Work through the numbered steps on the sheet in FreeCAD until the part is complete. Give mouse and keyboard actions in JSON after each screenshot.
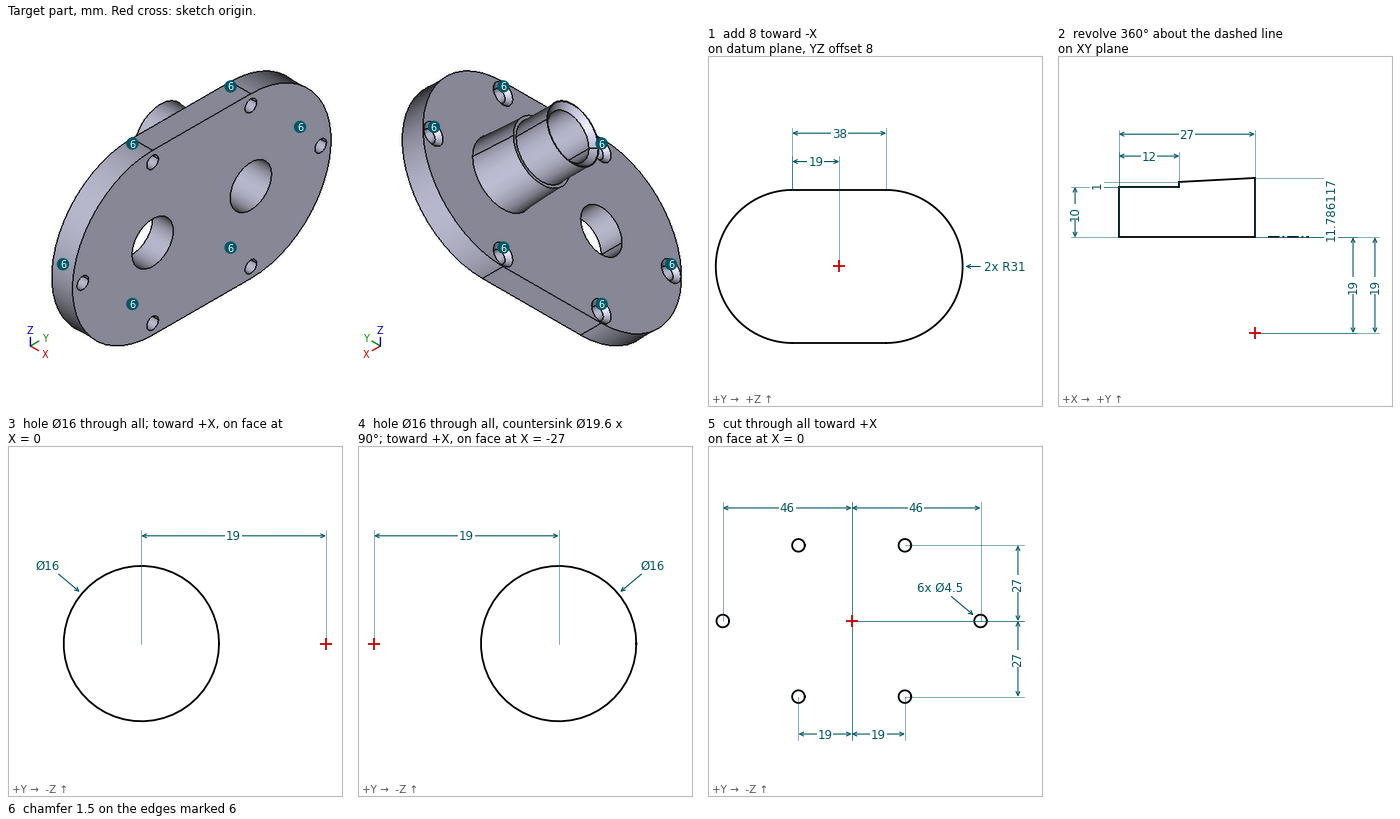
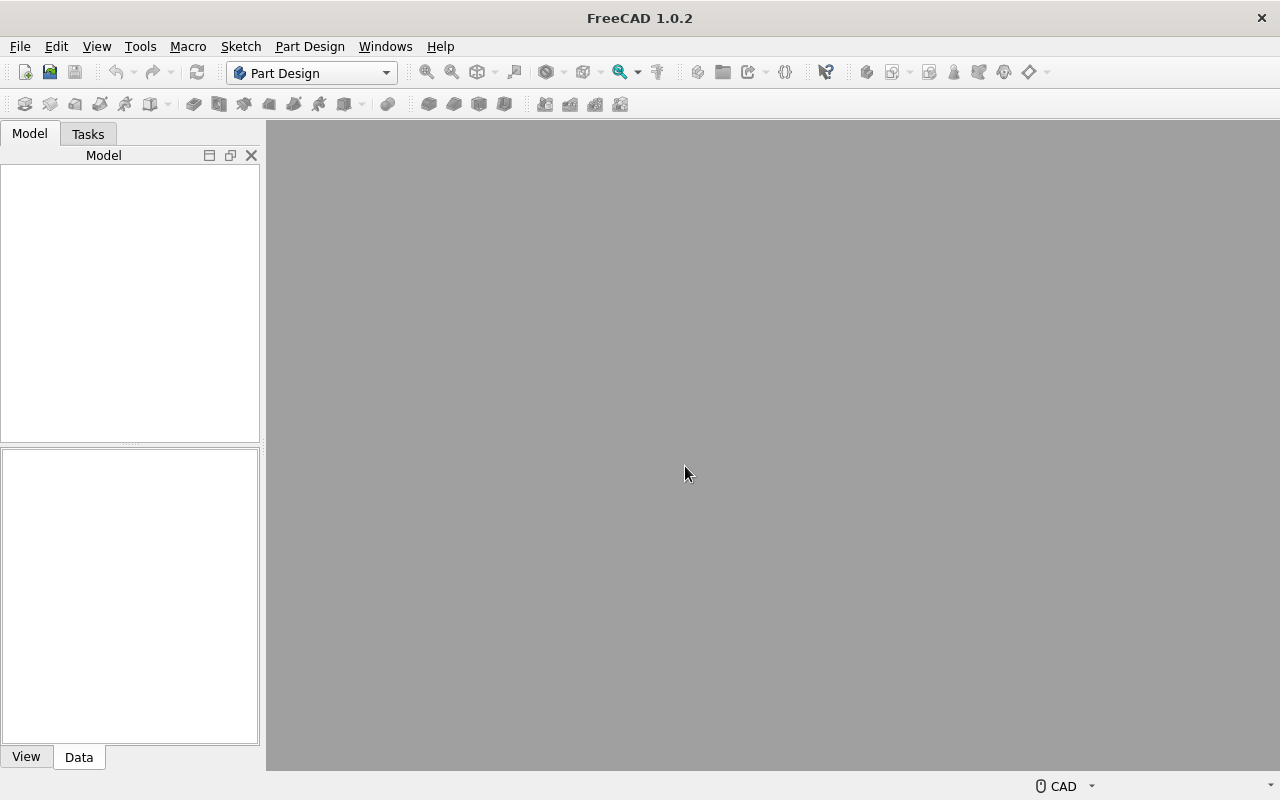
{"action": "key", "text": "ctrl+n"}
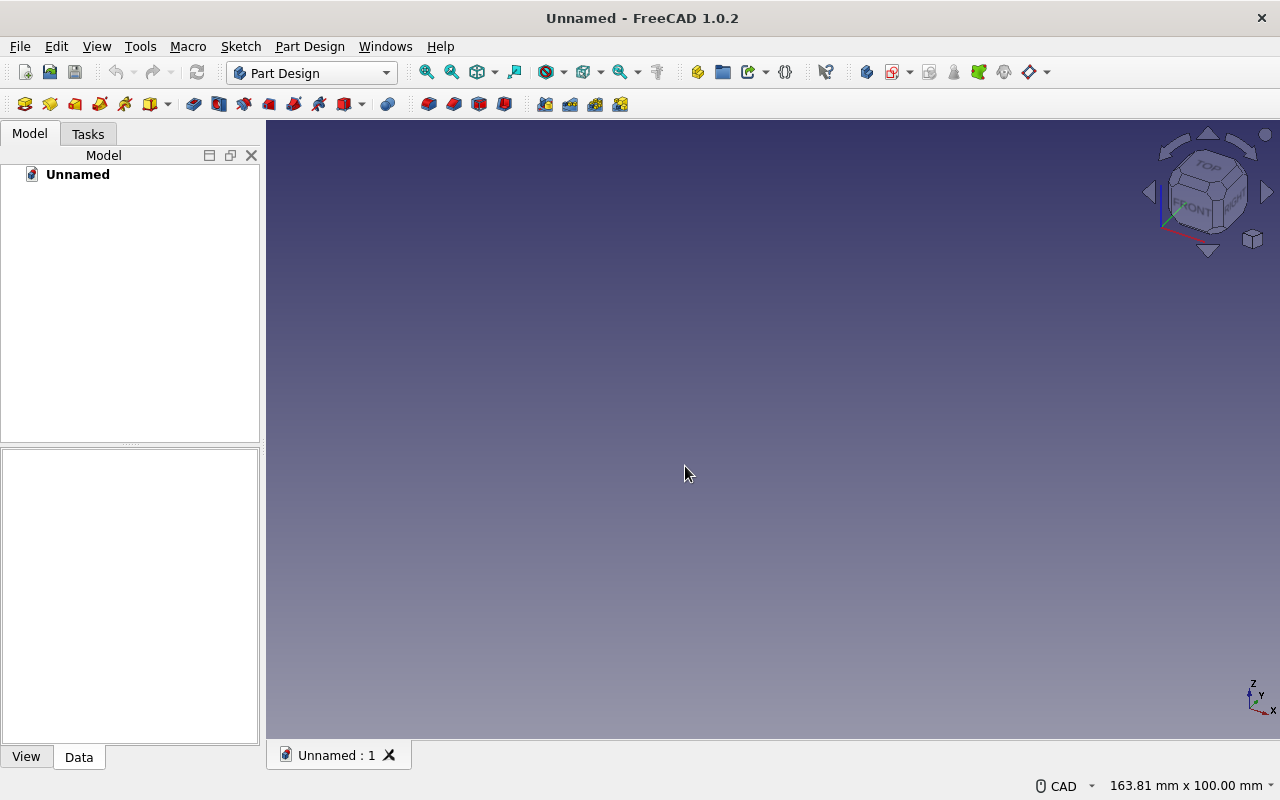
{"action": "left_click", "coordinate": [867, 72]}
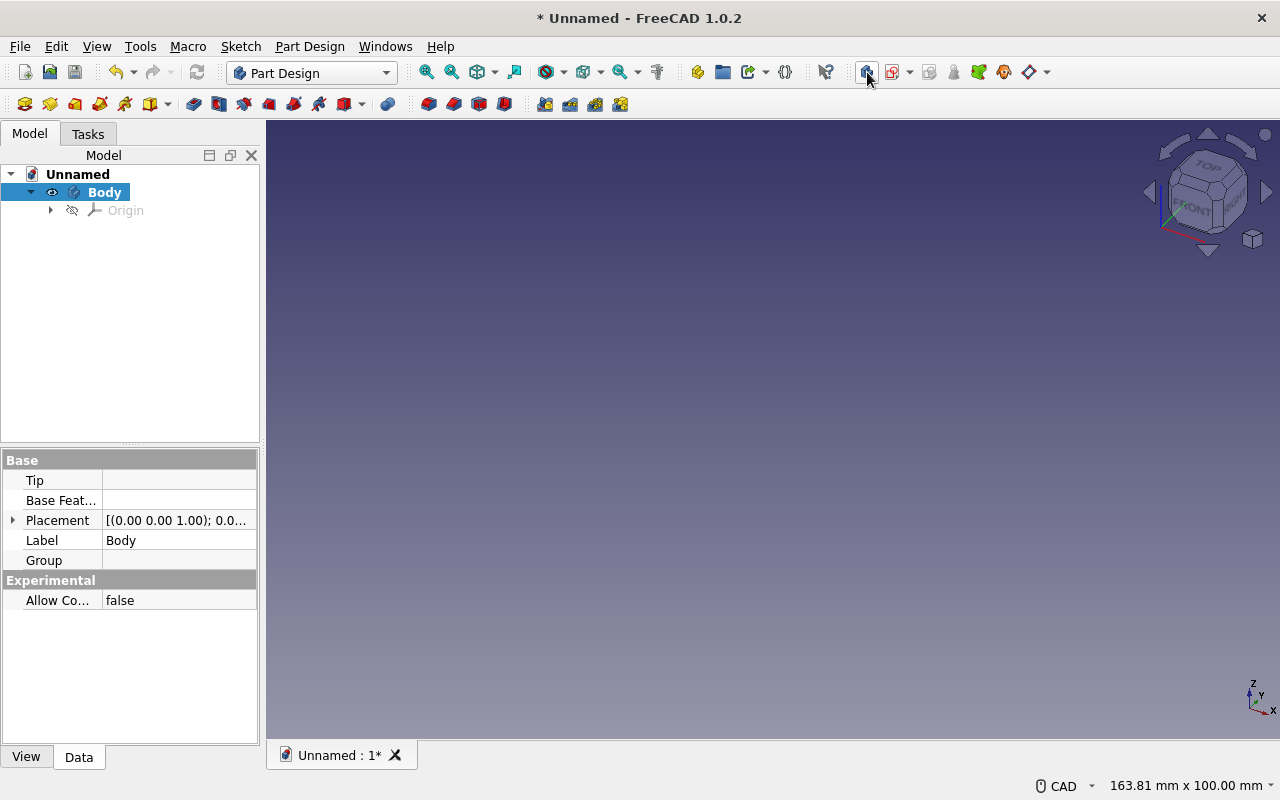
{"action": "left_click", "coordinate": [51, 210]}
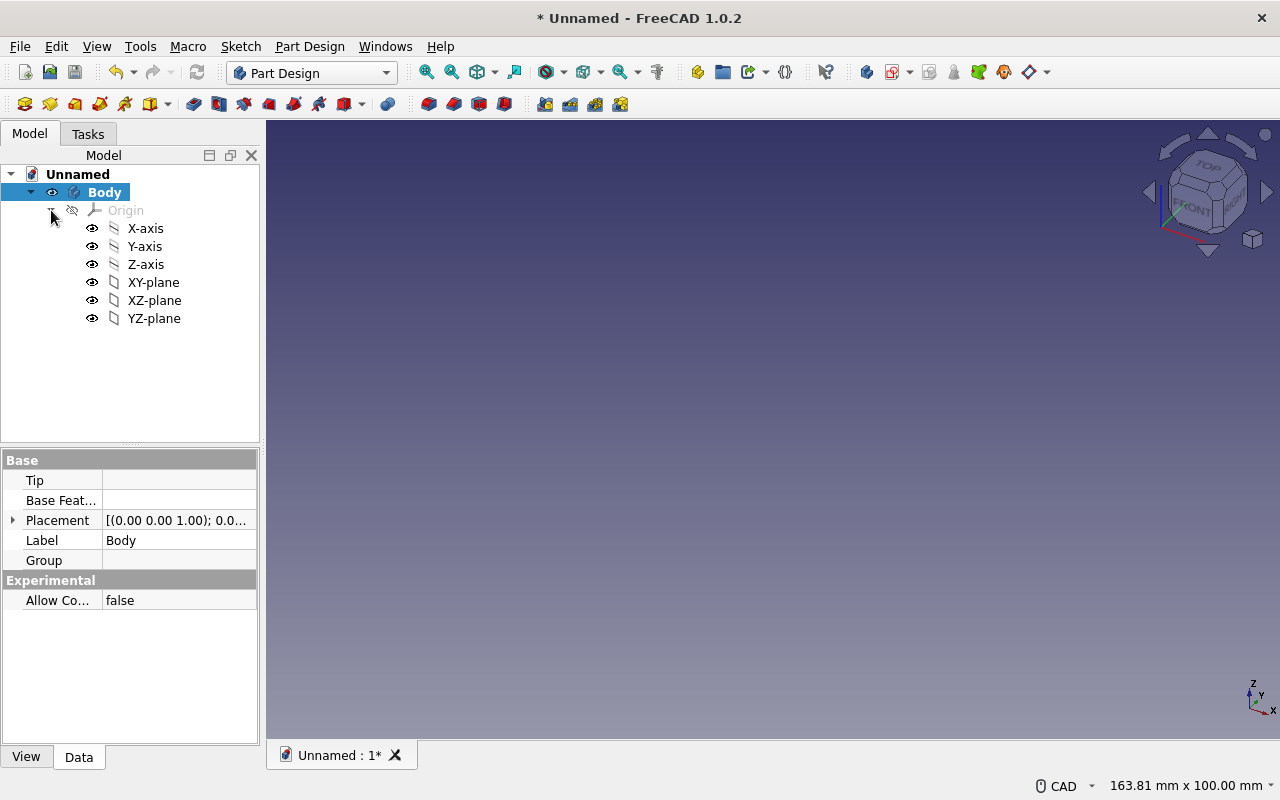
{"action": "left_click", "coordinate": [137, 318]}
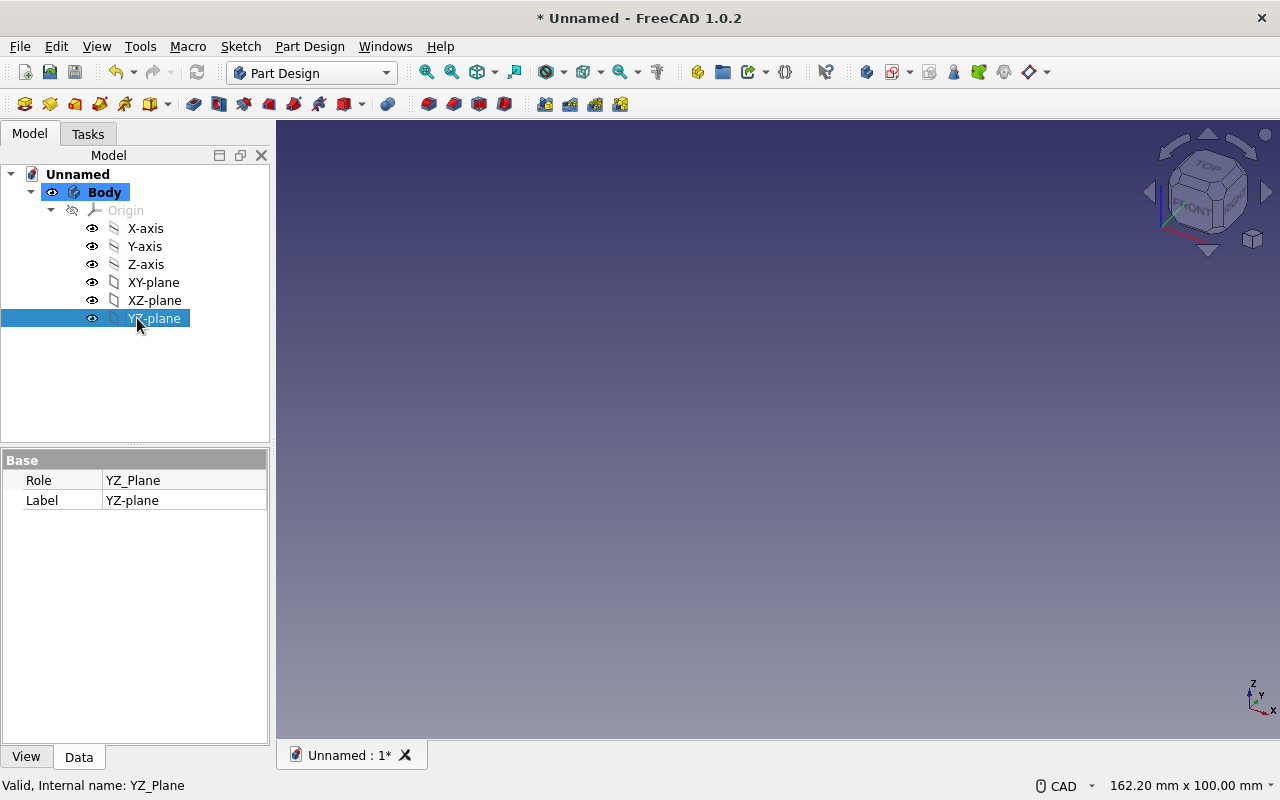
{"action": "left_click", "coordinate": [1028, 72]}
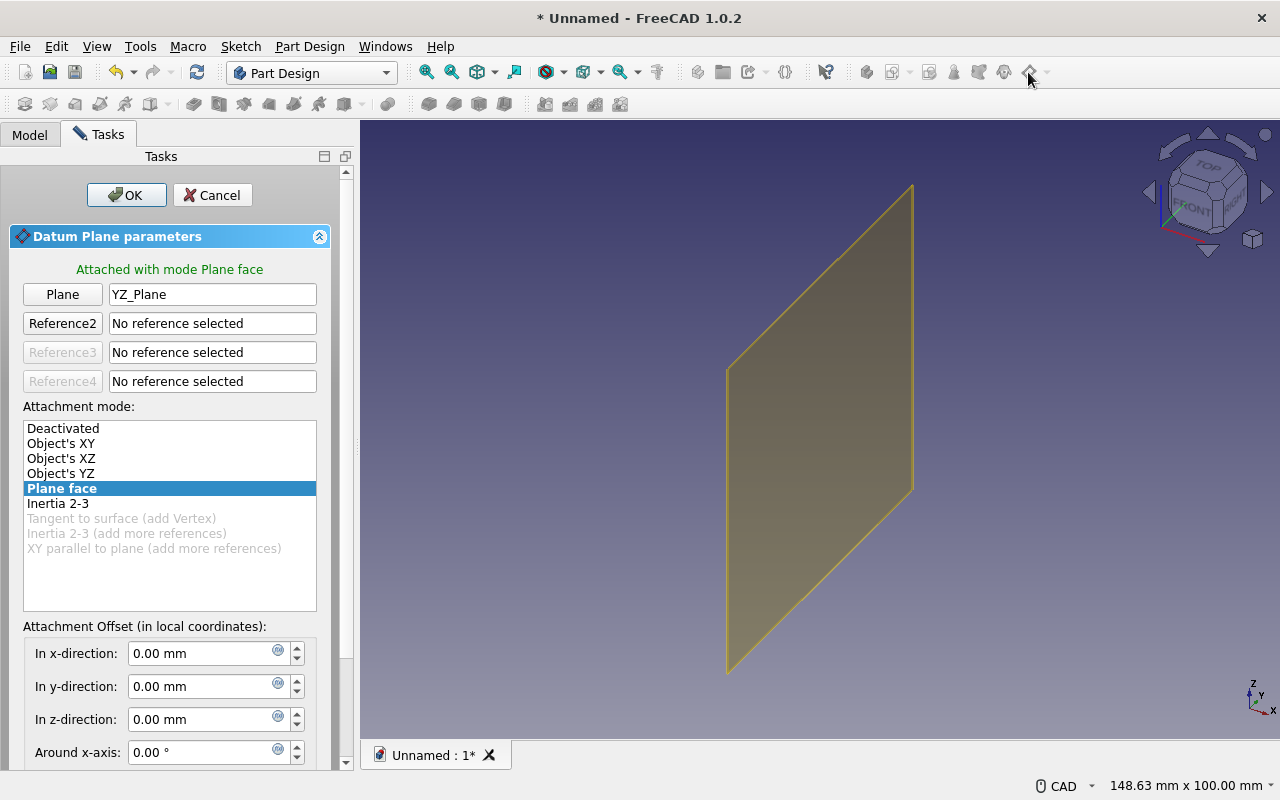
{"action": "triple_click", "coordinate": [210, 720]}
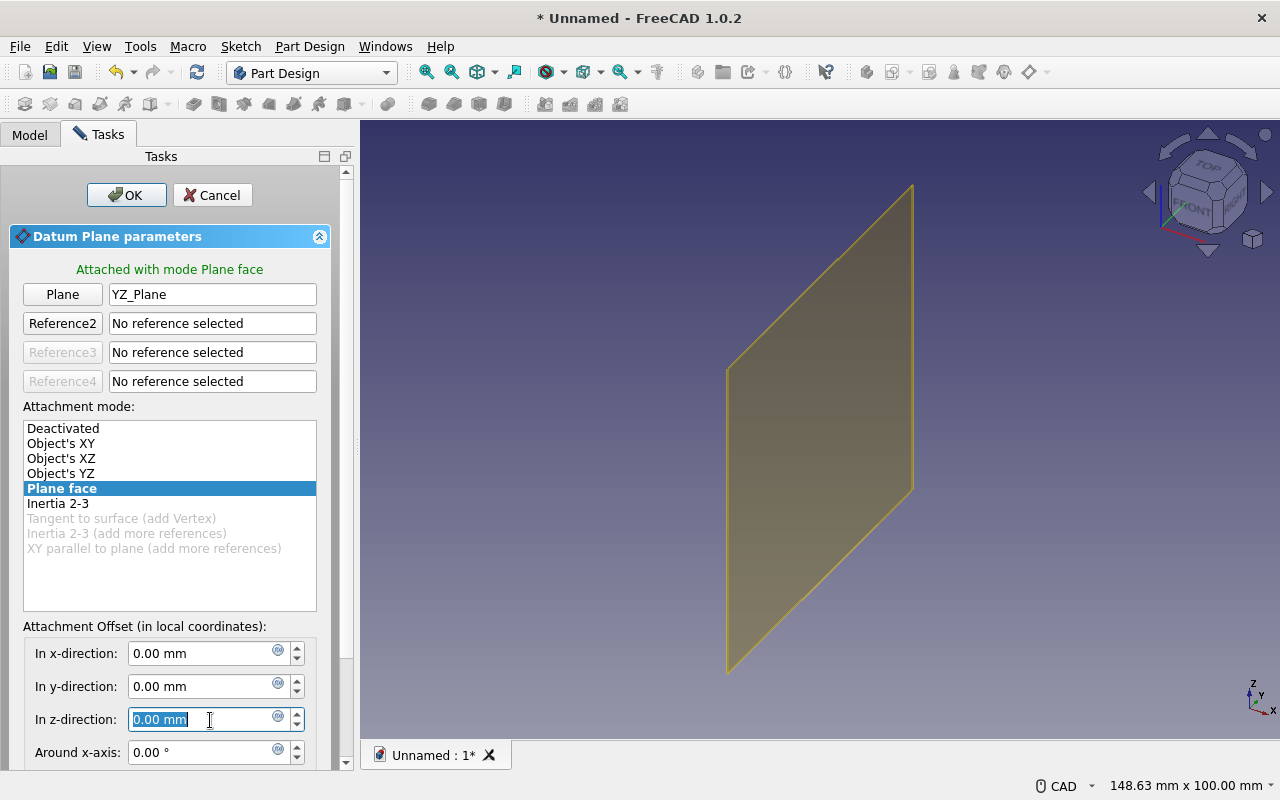
{"action": "type", "text": "8"}
{"action": "key", "text": "Tab"}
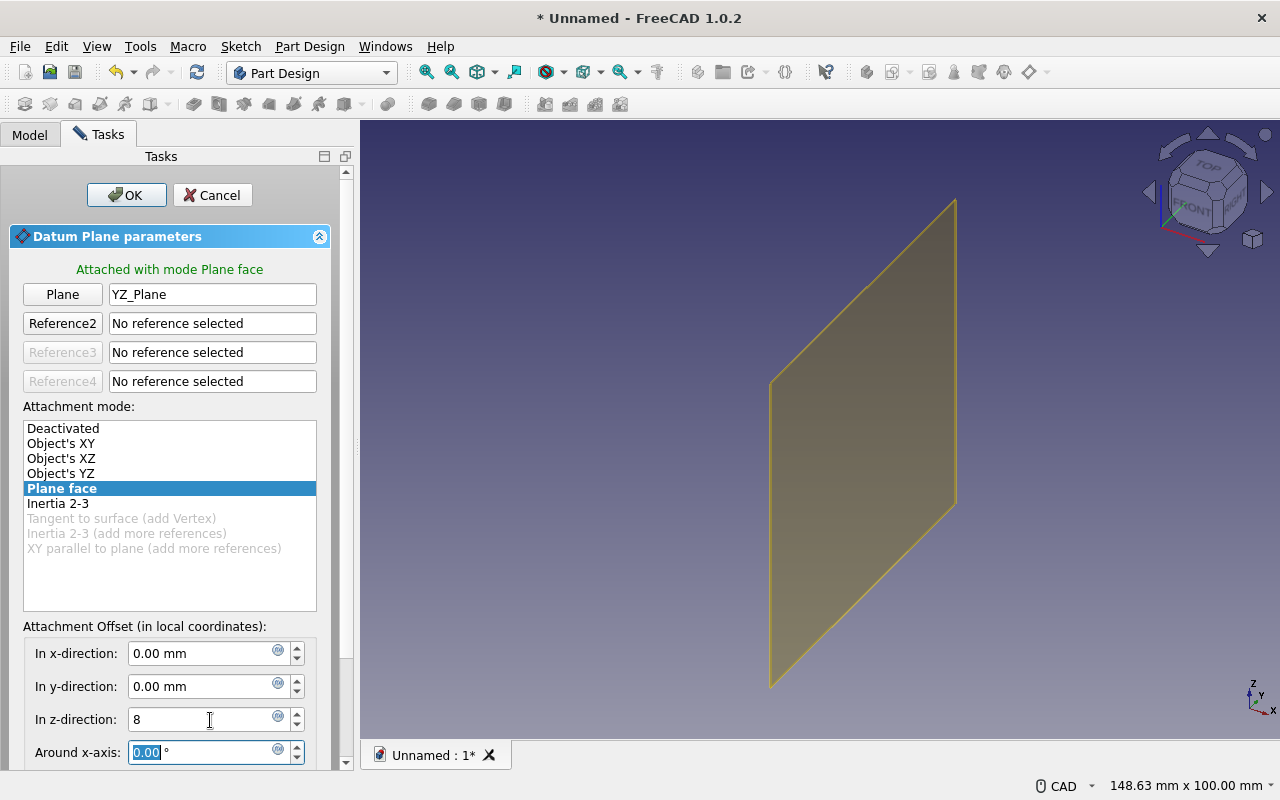
{"action": "left_click", "coordinate": [127, 195]}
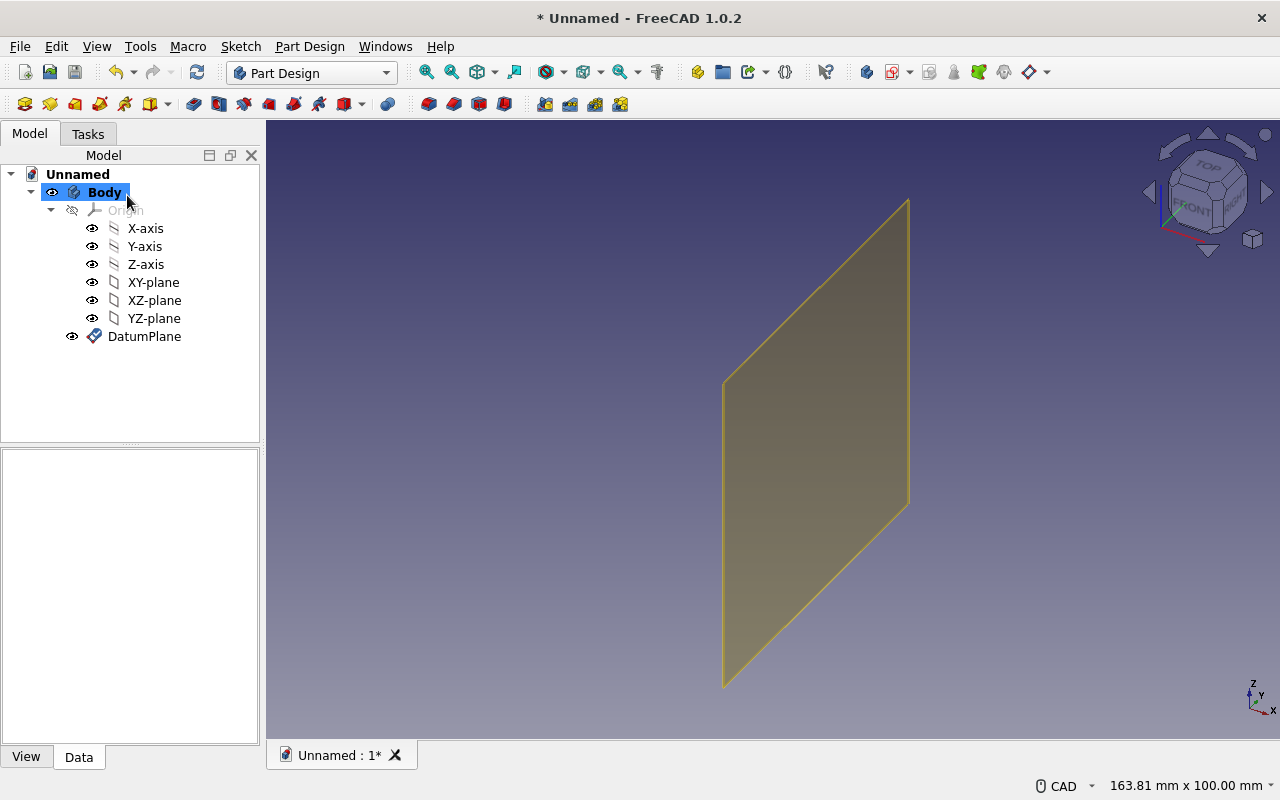
{"action": "left_click", "coordinate": [117, 336]}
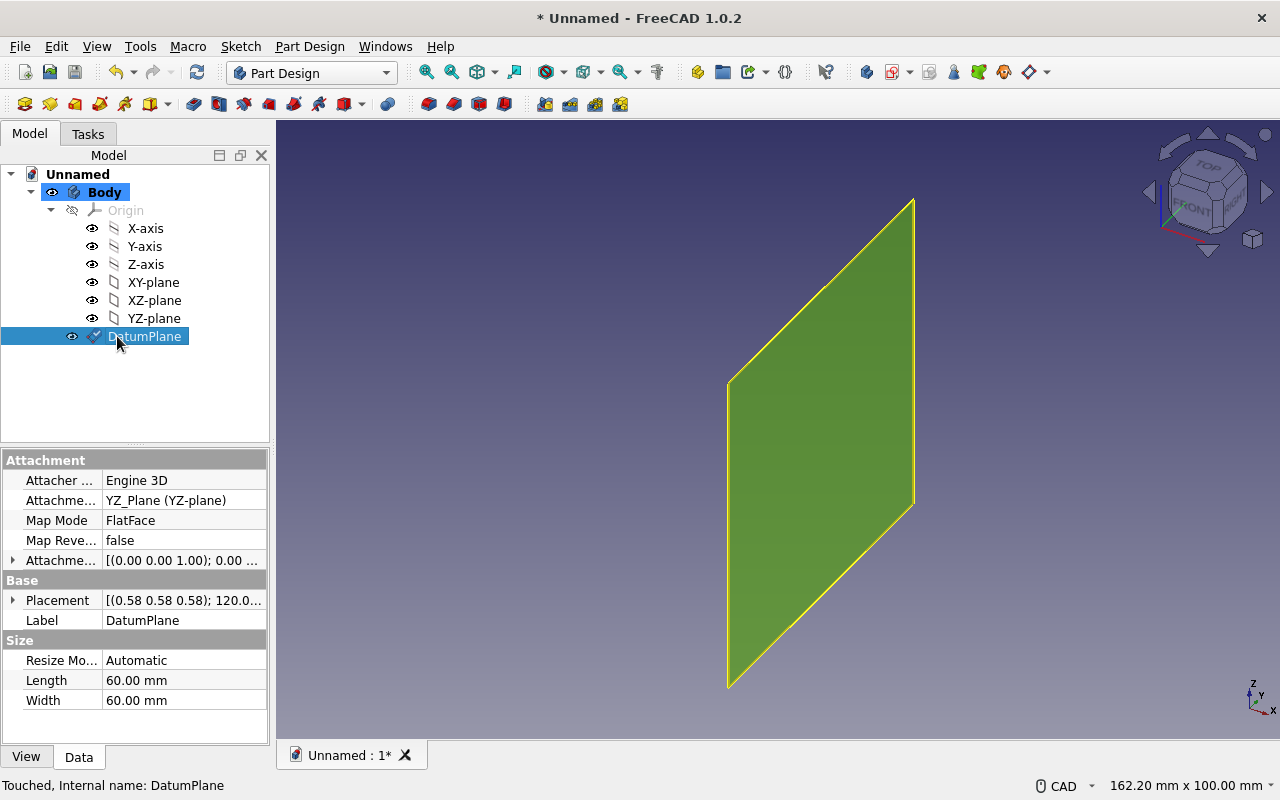
{"action": "left_click", "coordinate": [892, 72]}